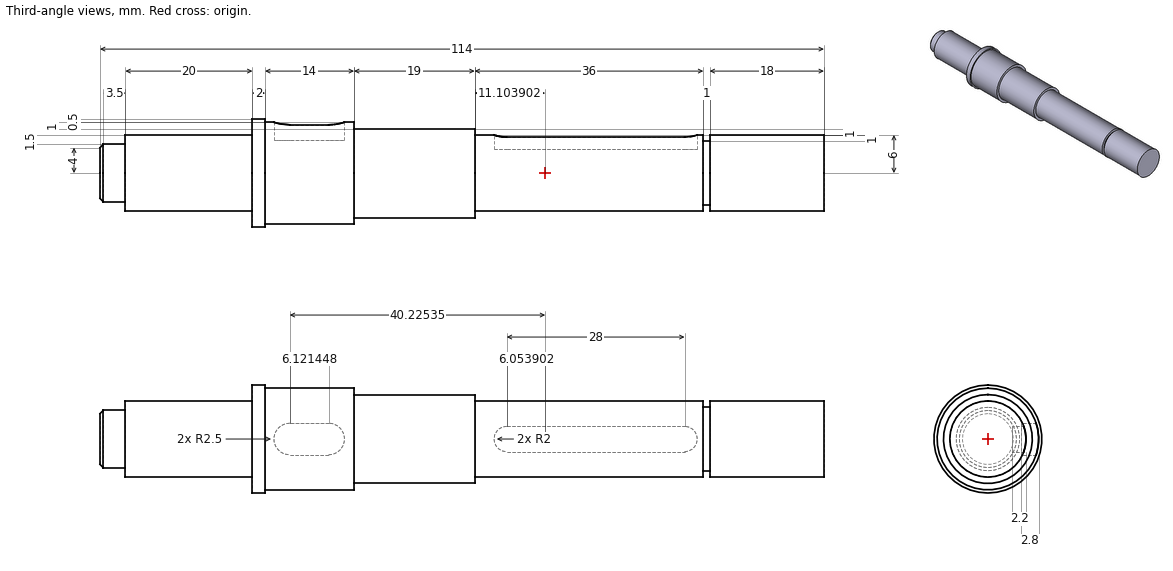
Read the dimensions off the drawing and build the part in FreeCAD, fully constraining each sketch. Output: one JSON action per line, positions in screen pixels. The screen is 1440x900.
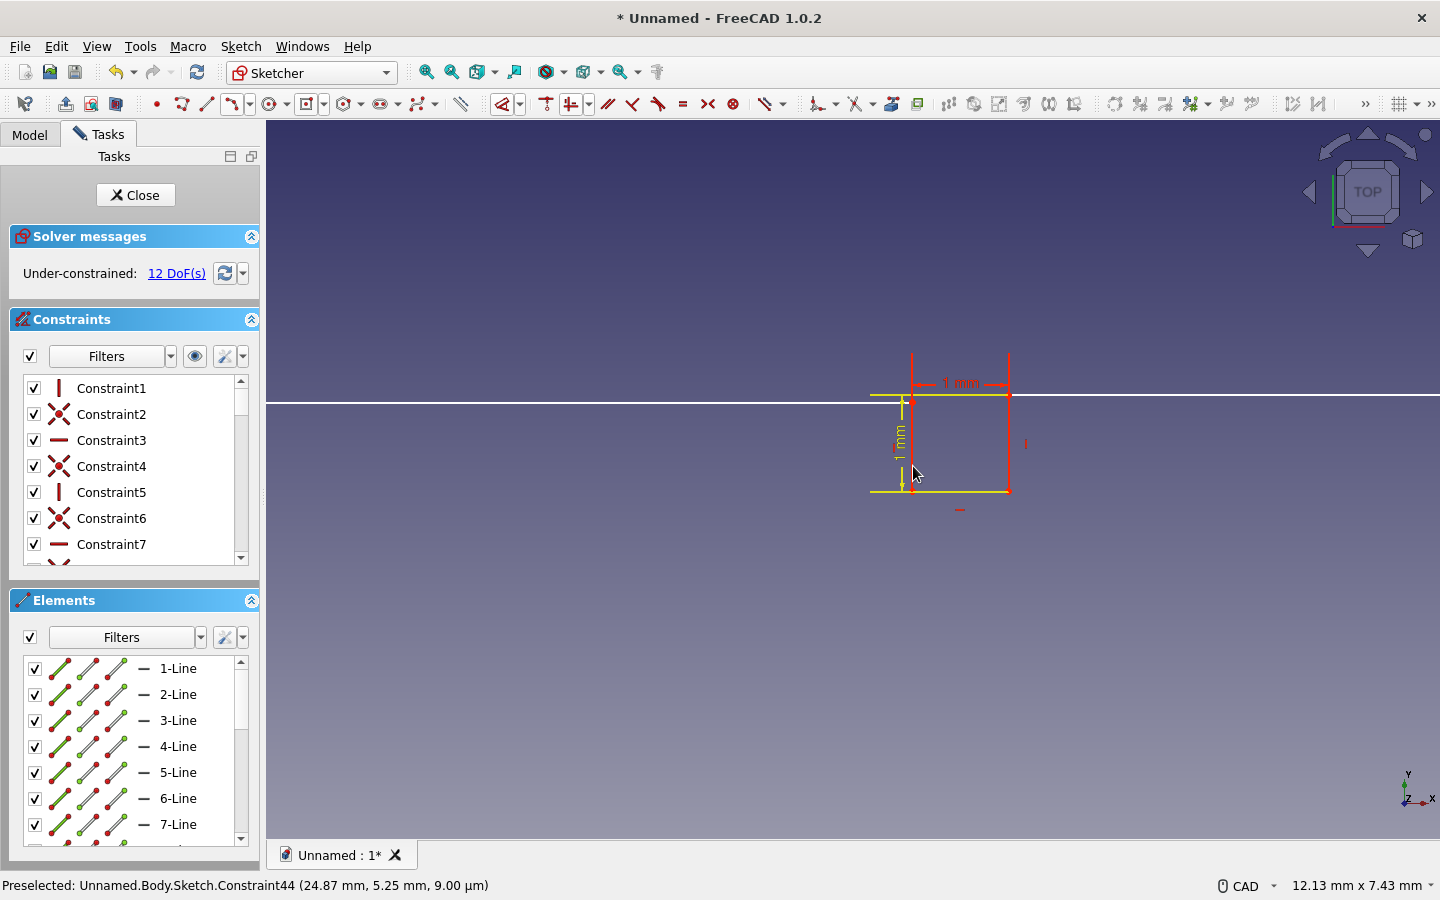
{"action": "left_click", "coordinate": [912, 465]}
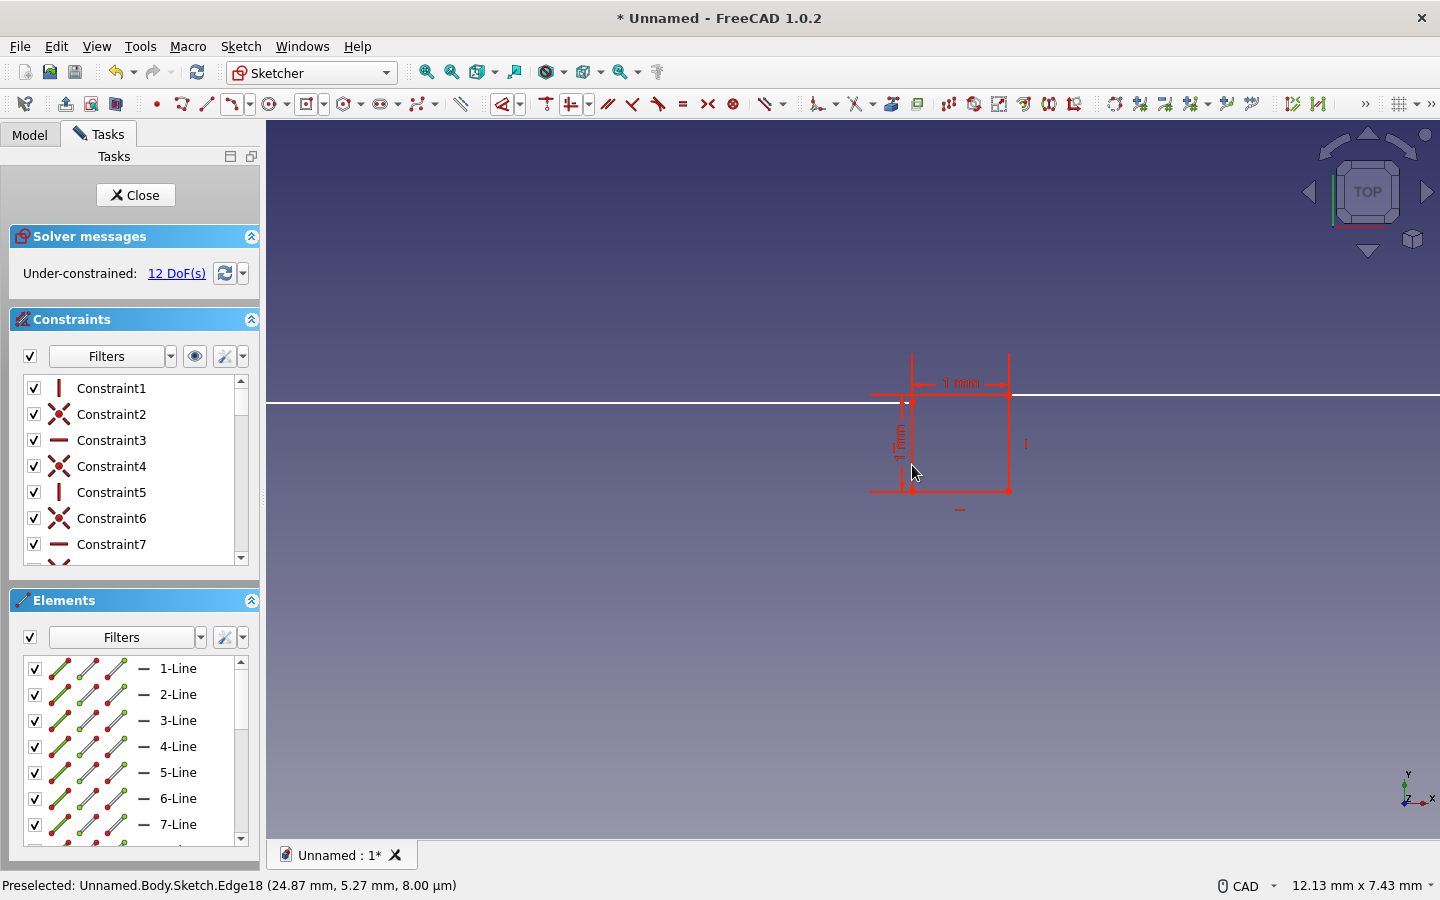
{"action": "key", "text": "i"}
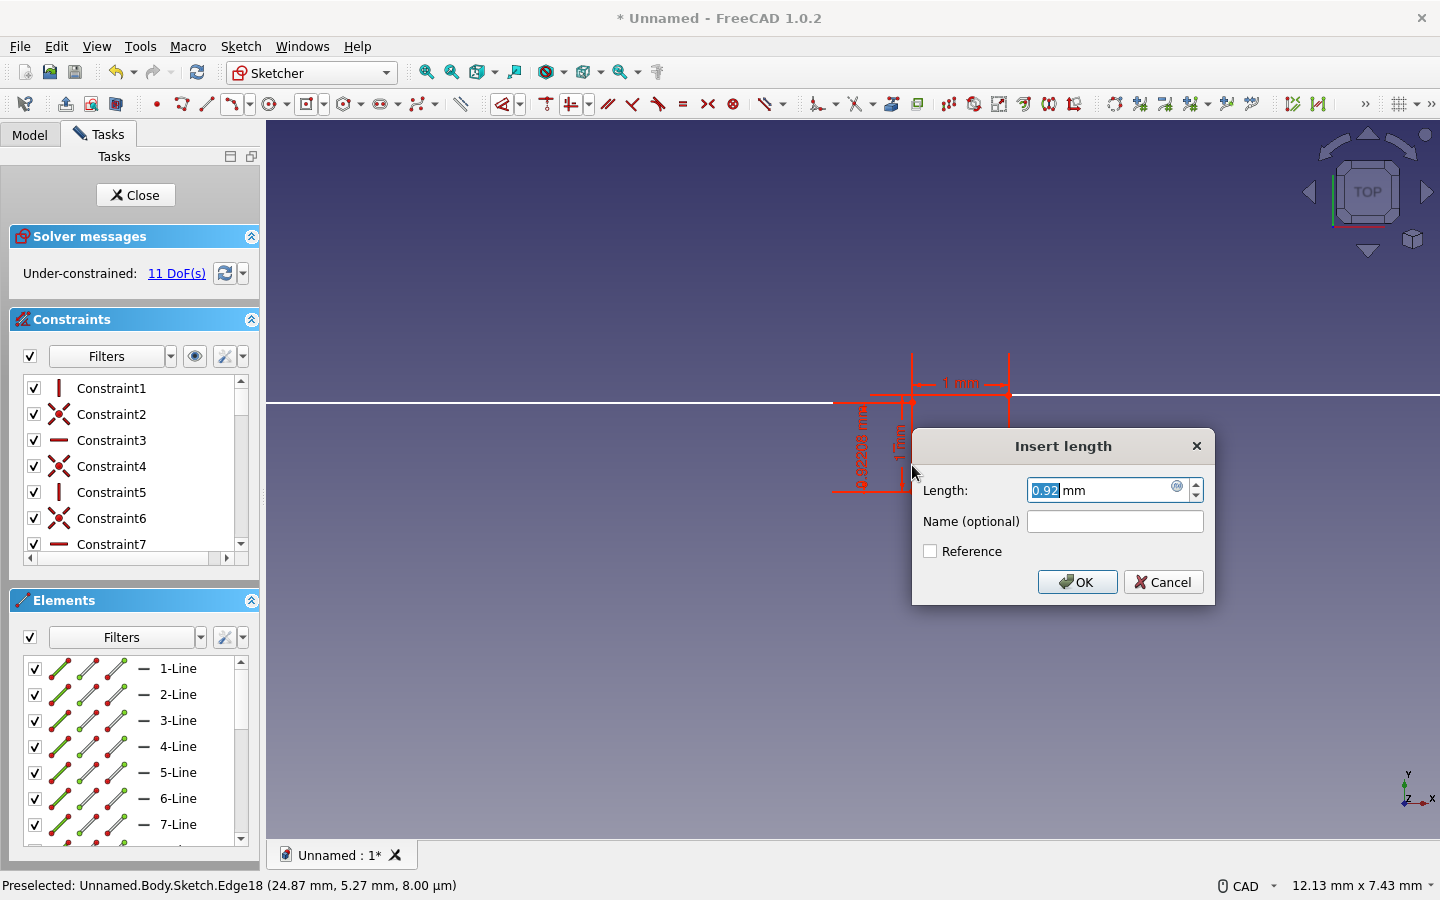
{"action": "type", "text": "1"}
{"action": "key", "text": "Return"}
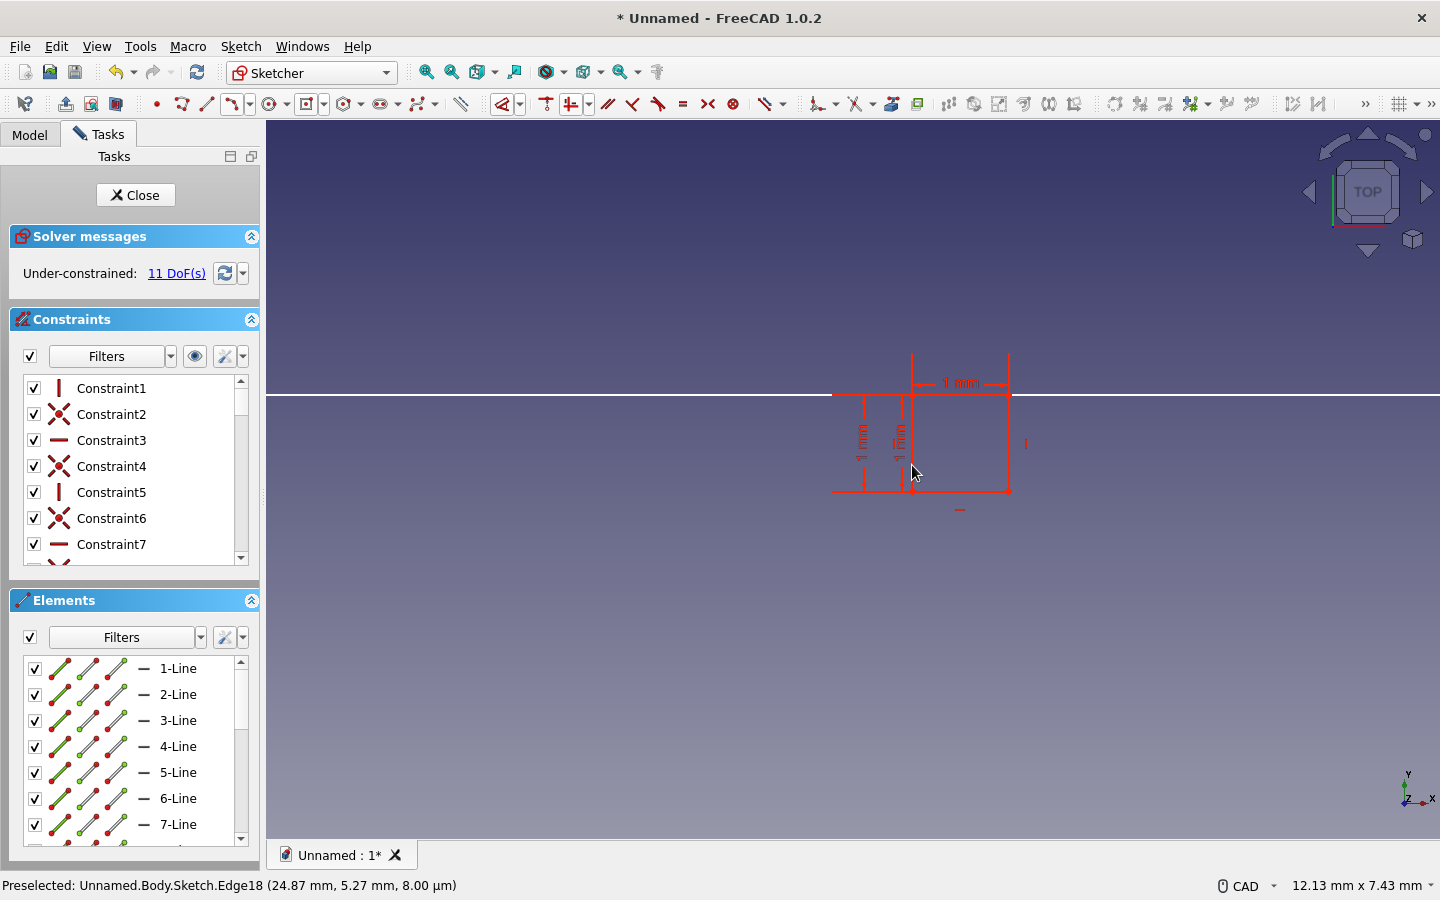
{"action": "scroll", "coordinate": [1014, 474], "scroll_direction": "down", "scroll_amount": 14}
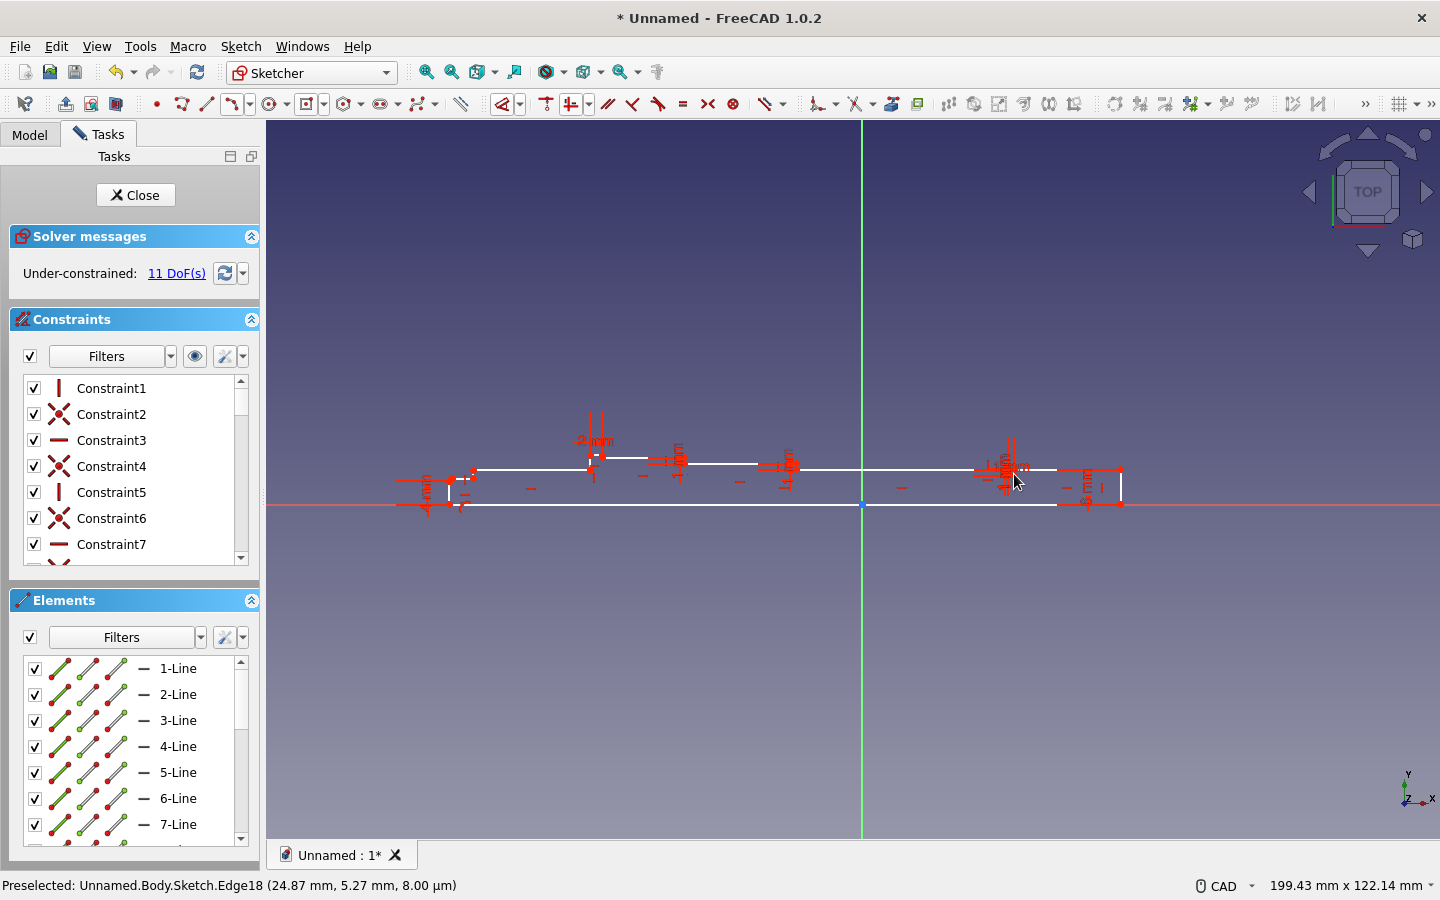
{"action": "left_click", "coordinate": [763, 464]}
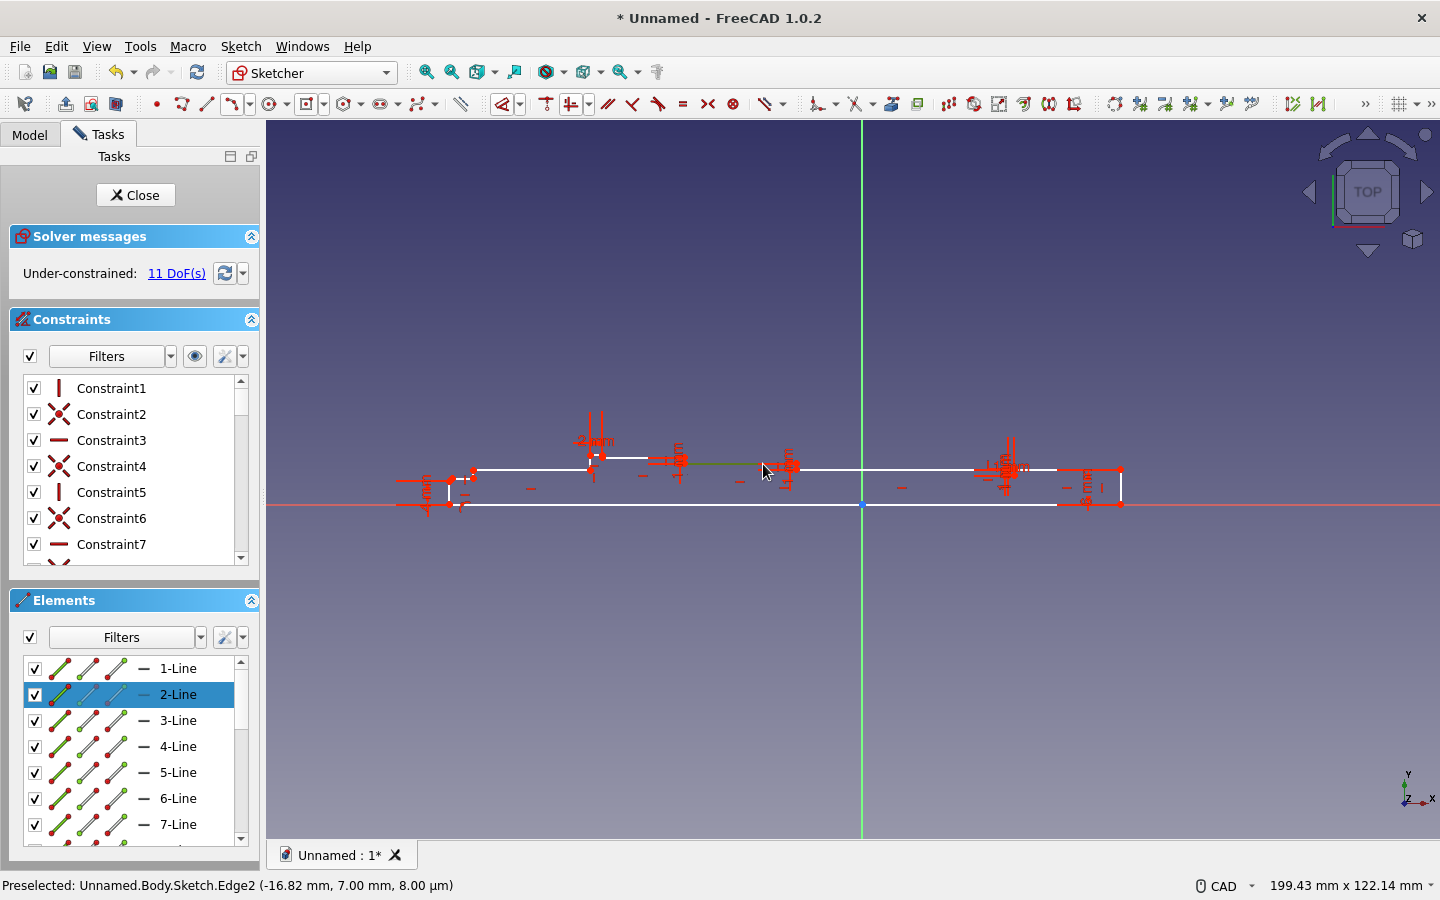
{"action": "key", "text": "l"}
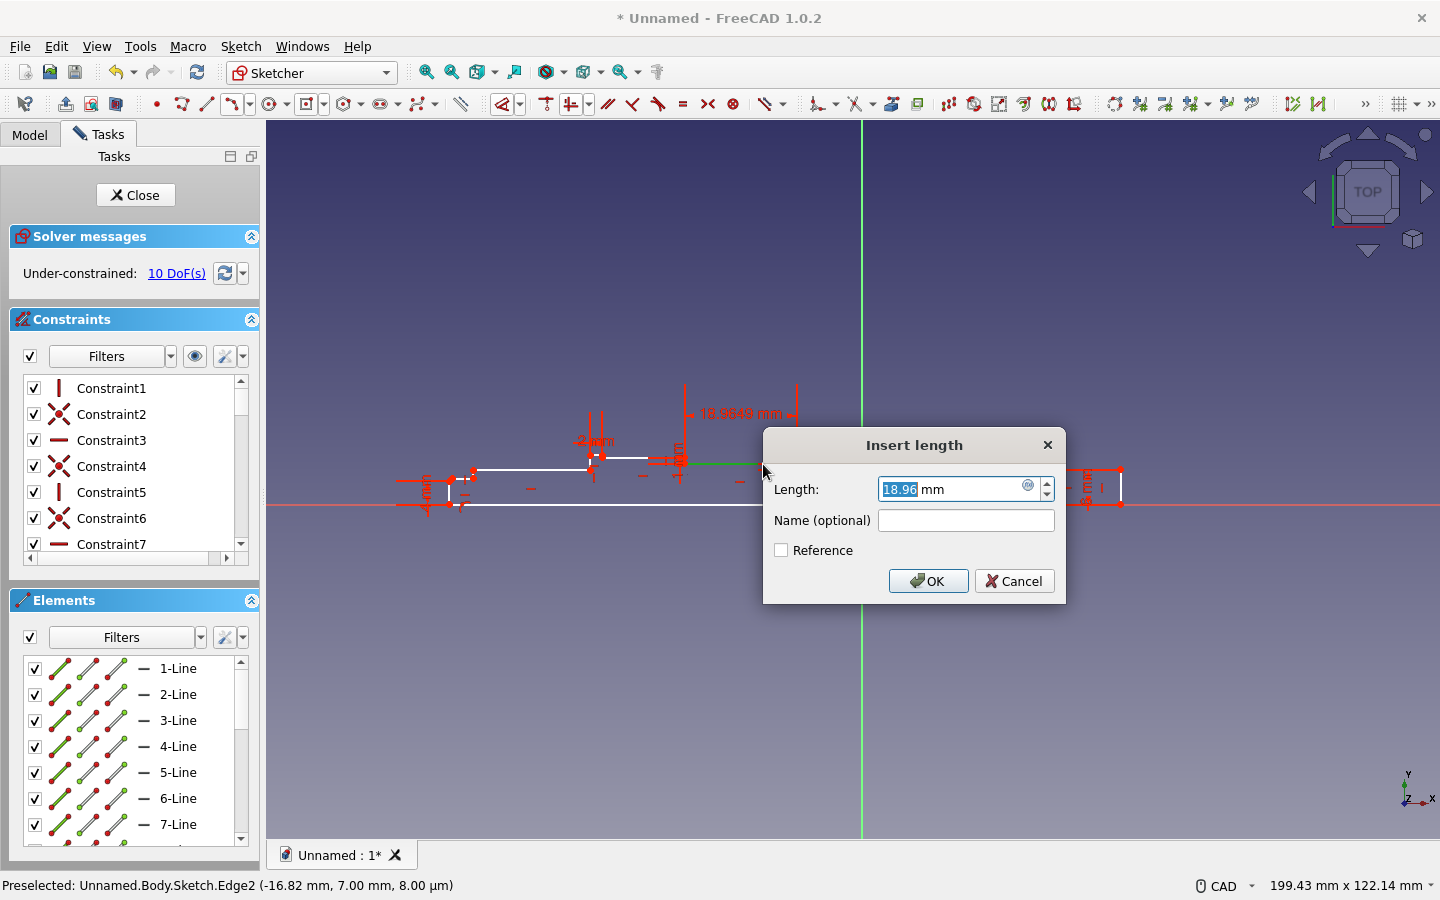
{"action": "type", "text": "19"}
{"action": "key", "text": "Return"}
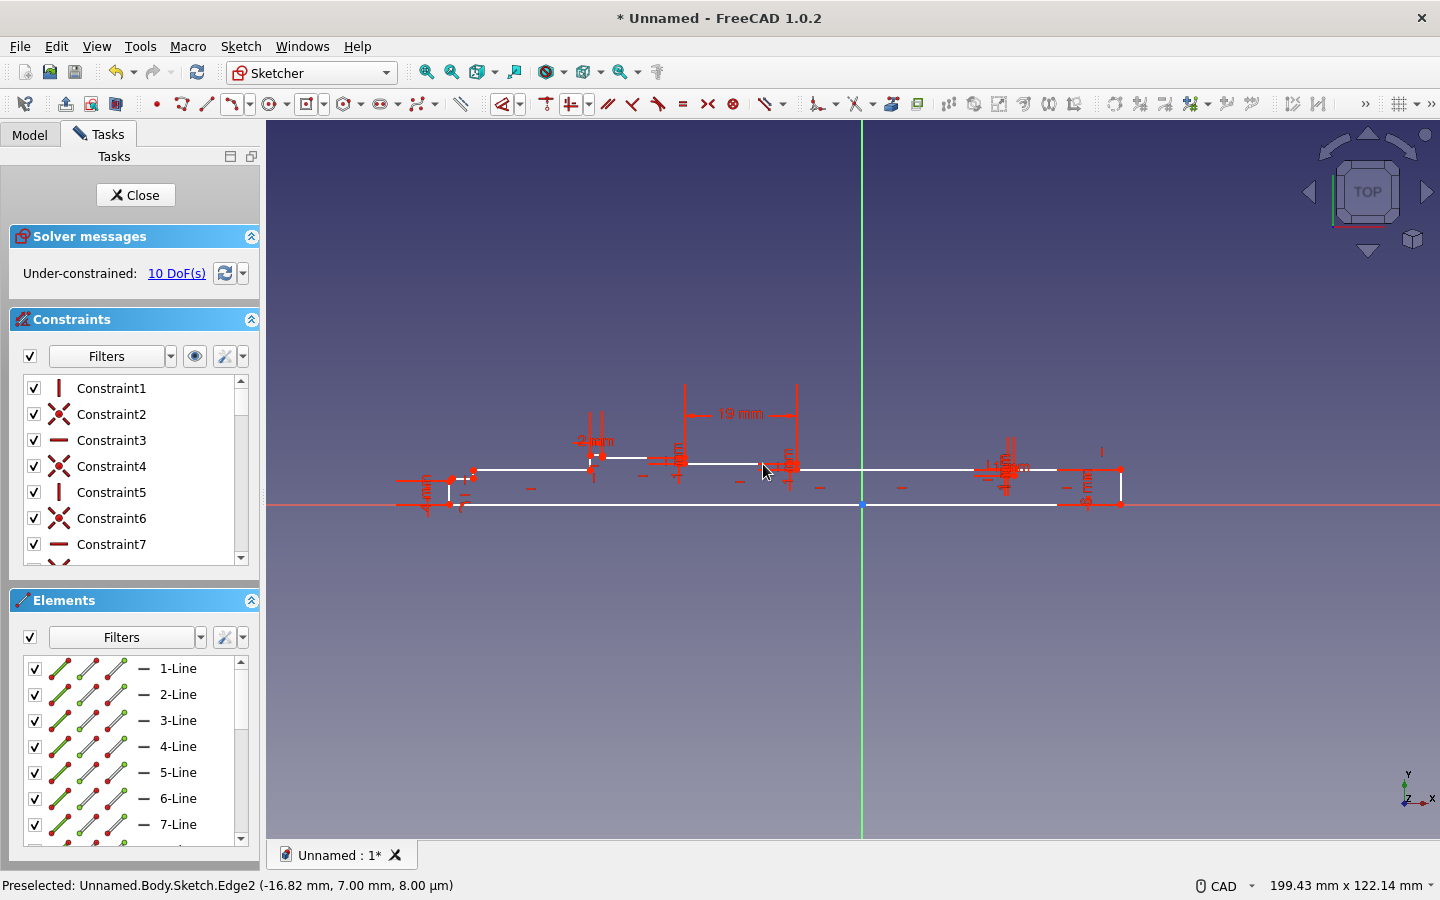
{"action": "left_click", "coordinate": [660, 458]}